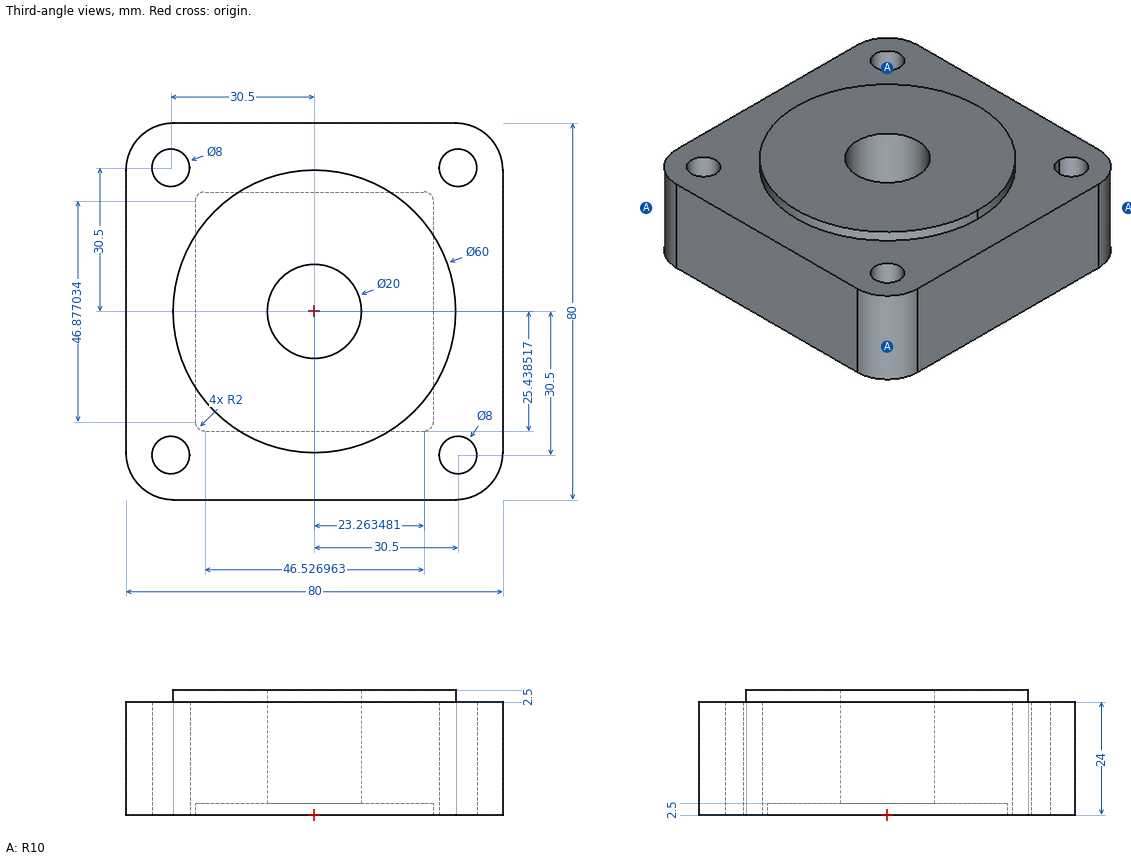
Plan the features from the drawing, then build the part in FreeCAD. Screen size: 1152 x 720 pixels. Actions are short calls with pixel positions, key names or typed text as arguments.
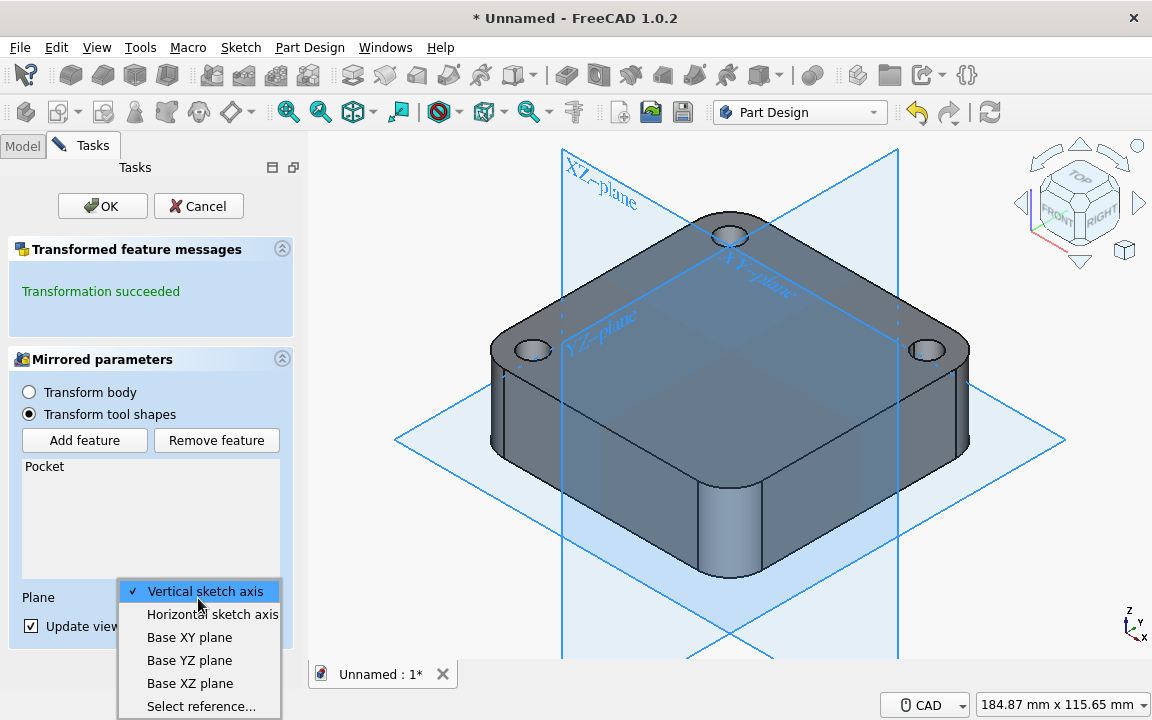
click(198, 660)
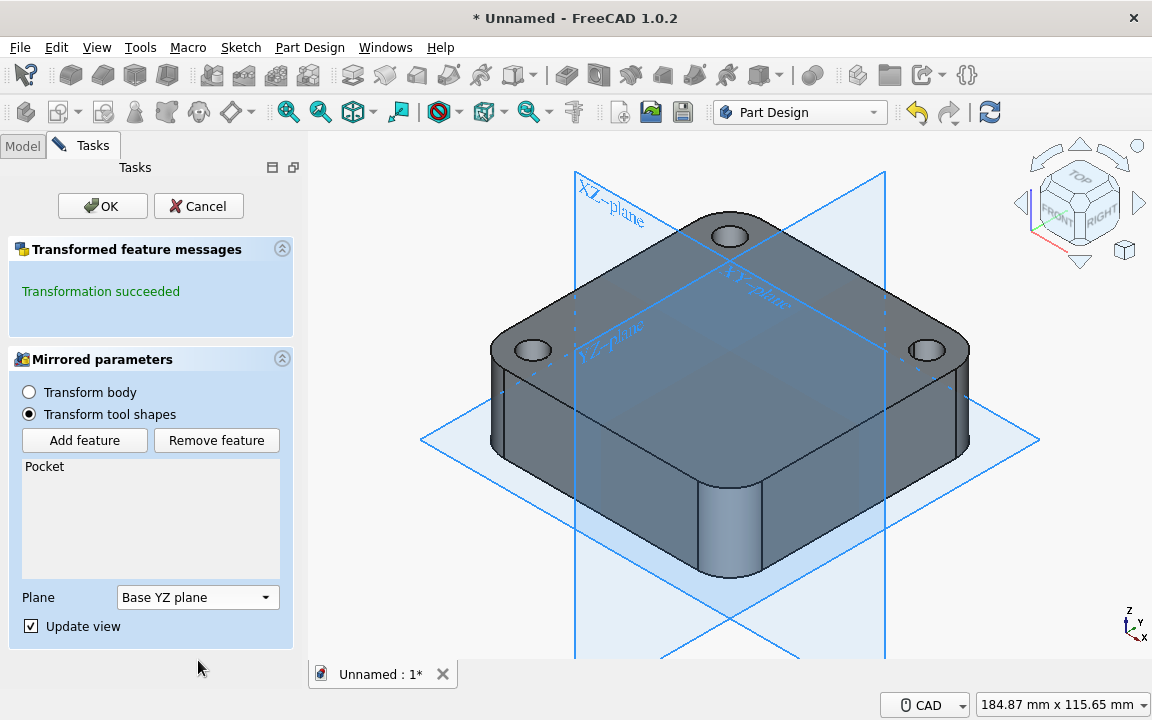
click(103, 206)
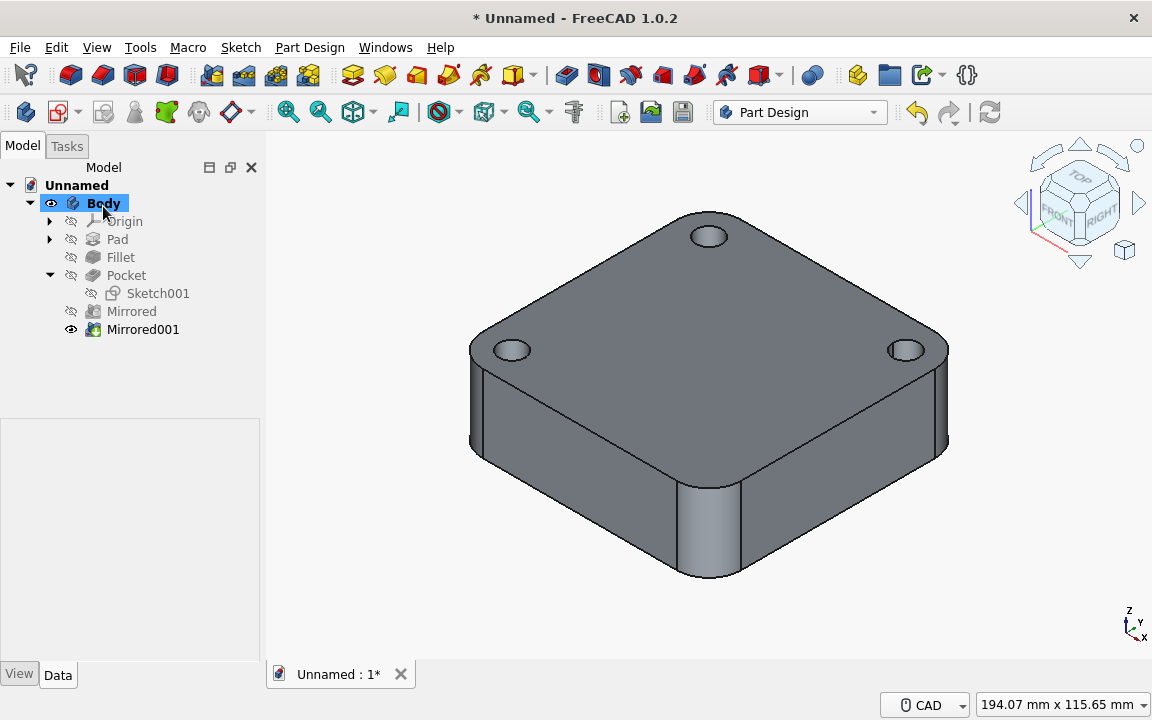
click(709, 349)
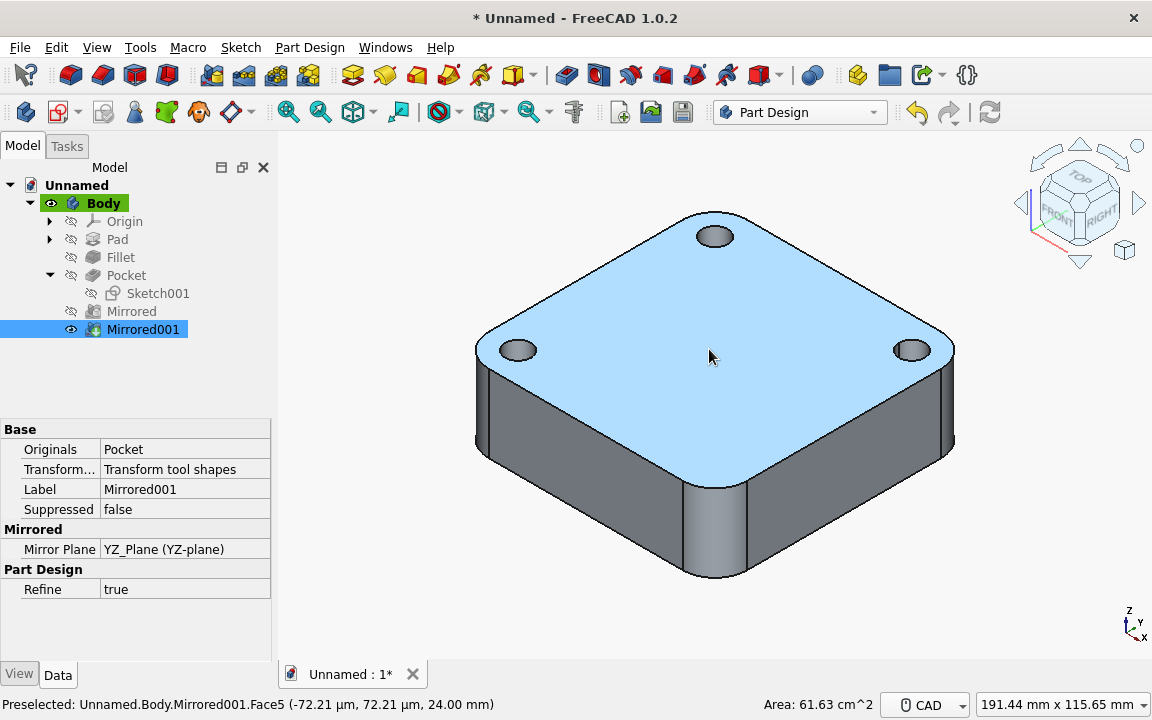
click(58, 112)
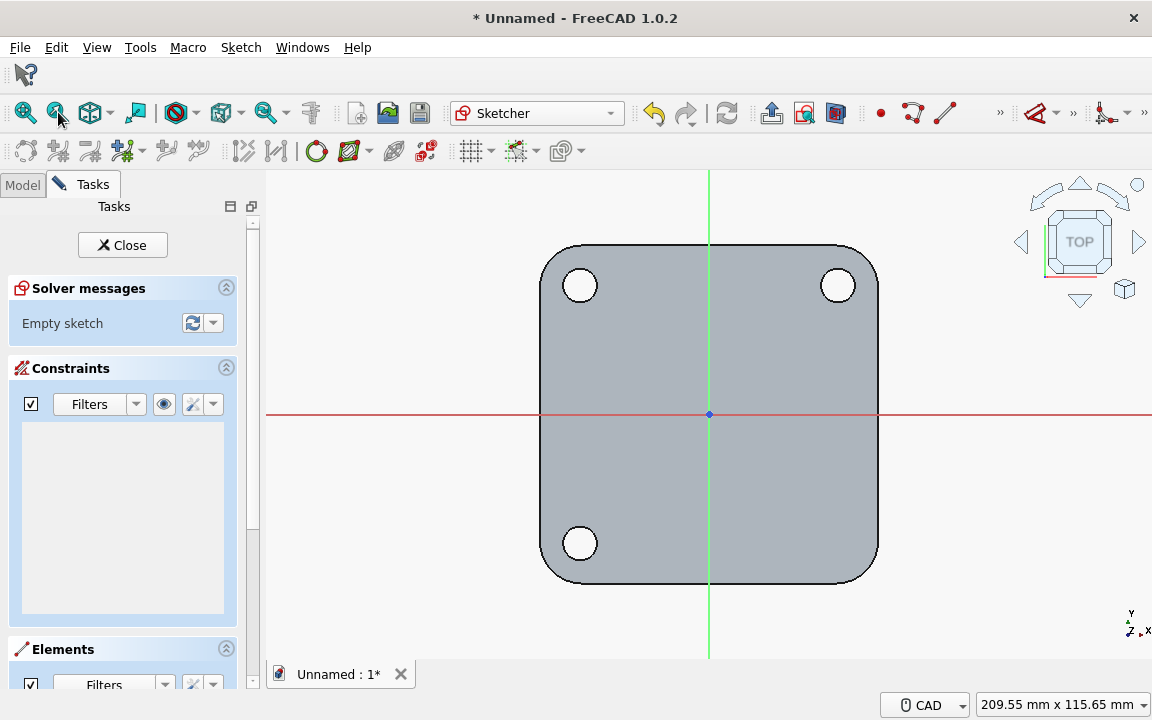
scroll(863, 560, up, 11)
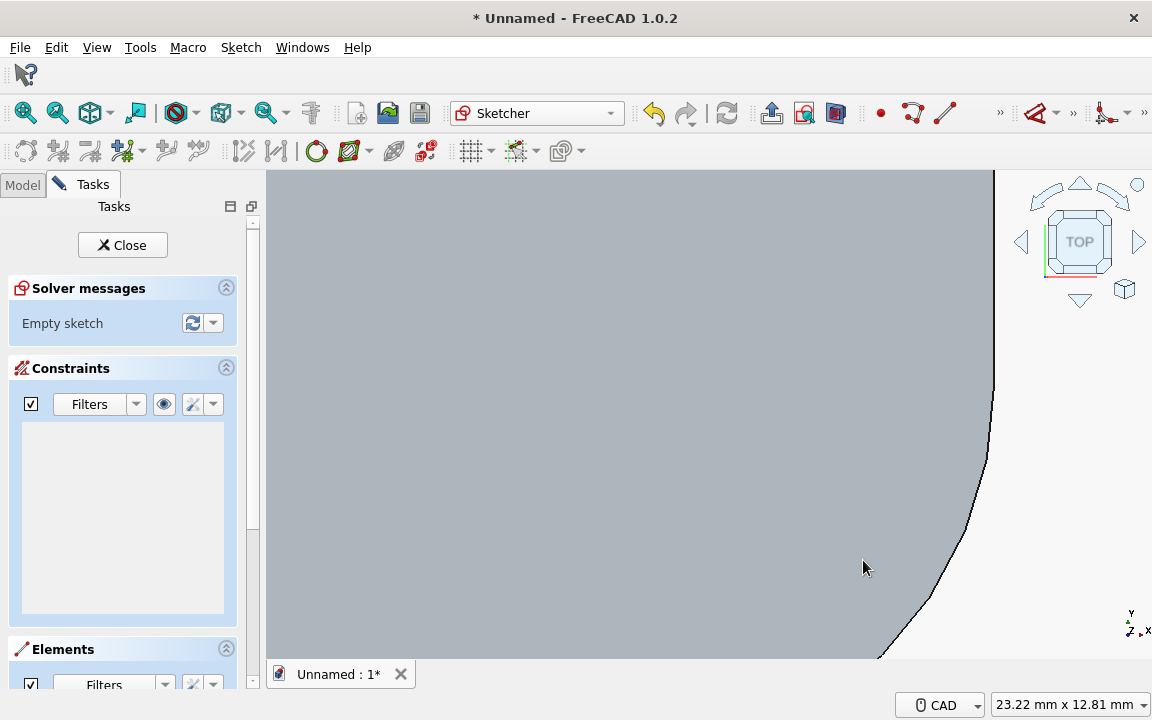
key(g)
key(c)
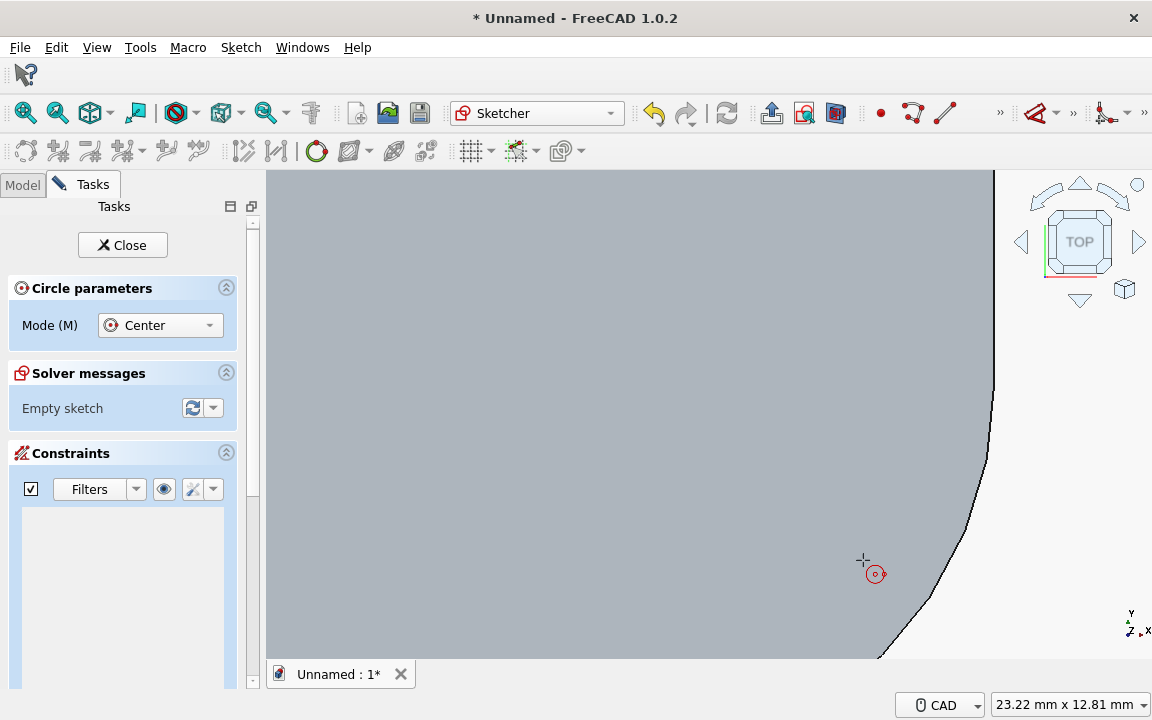
click(632, 404)
click(740, 296)
key(Escape)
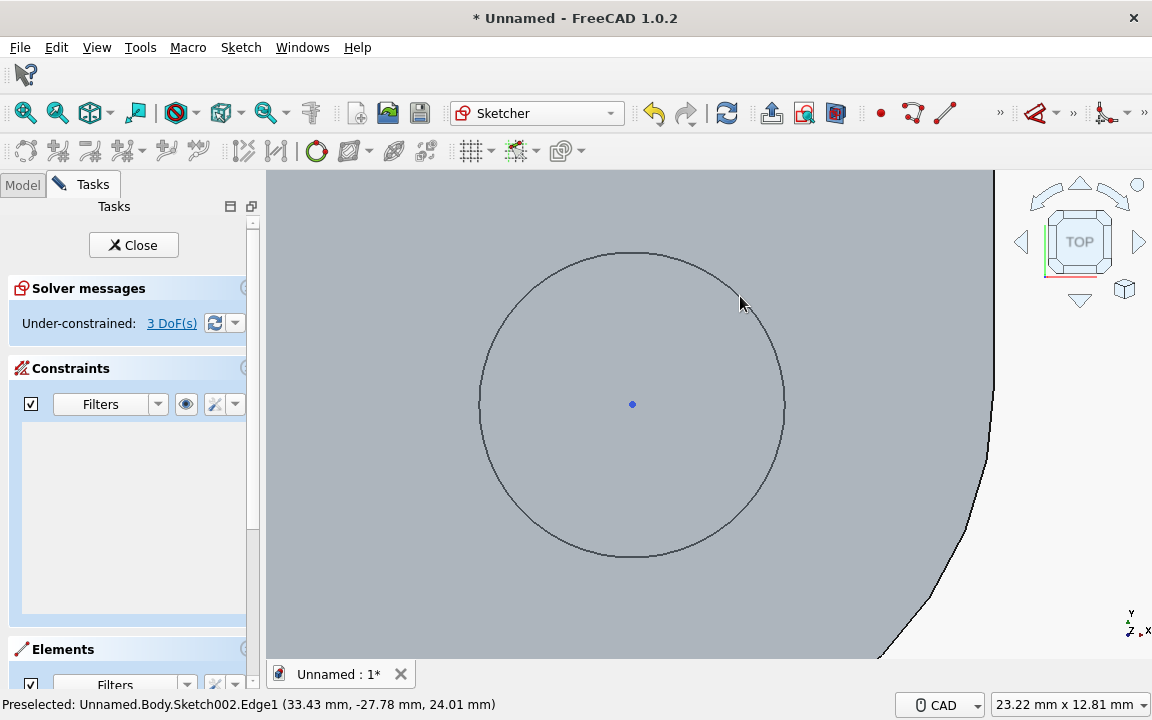
click(1036, 114)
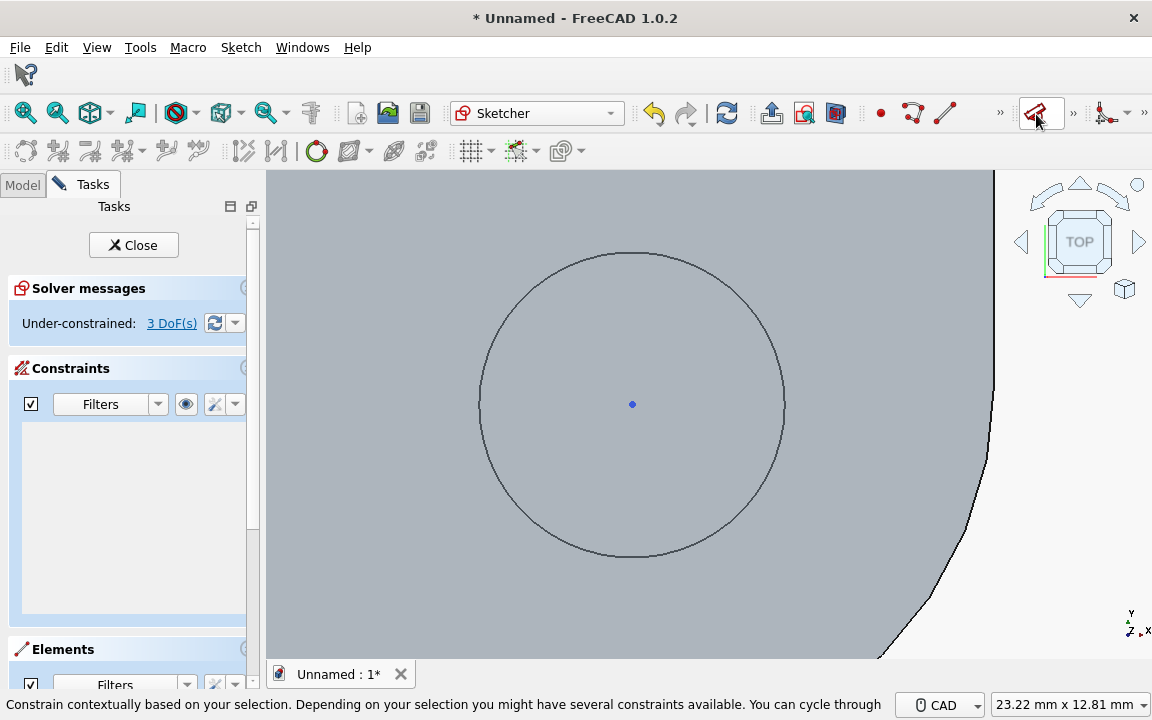
click(740, 297)
click(763, 274)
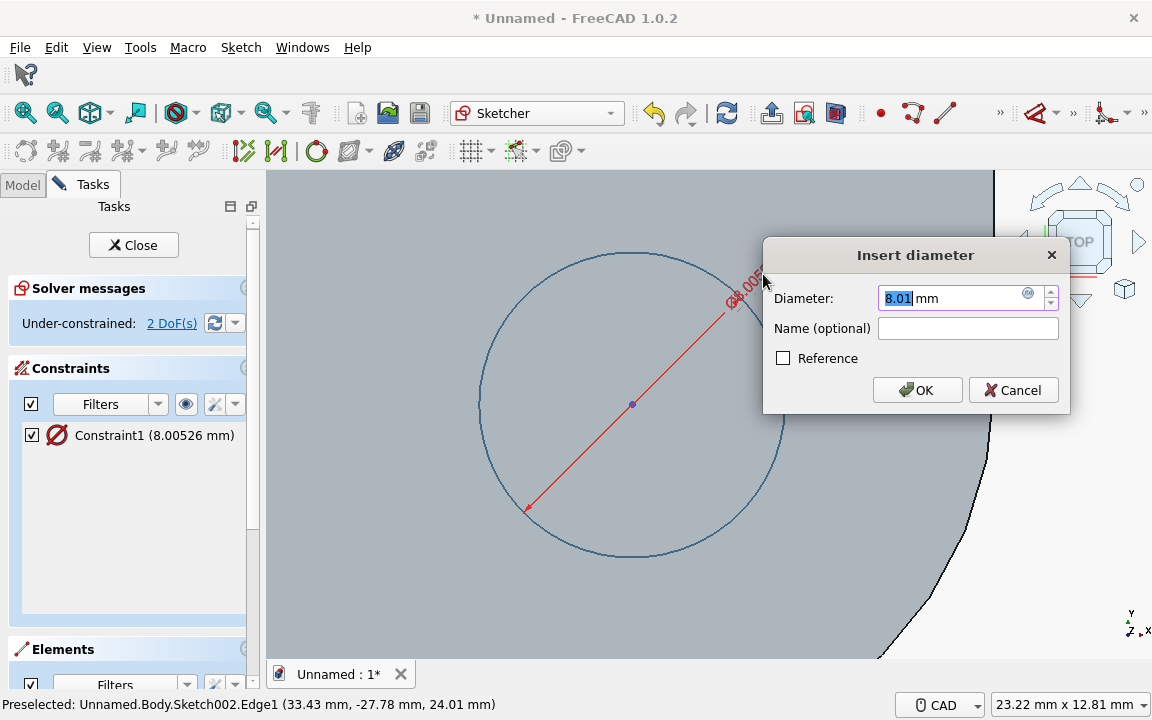
text(8)
key(Return)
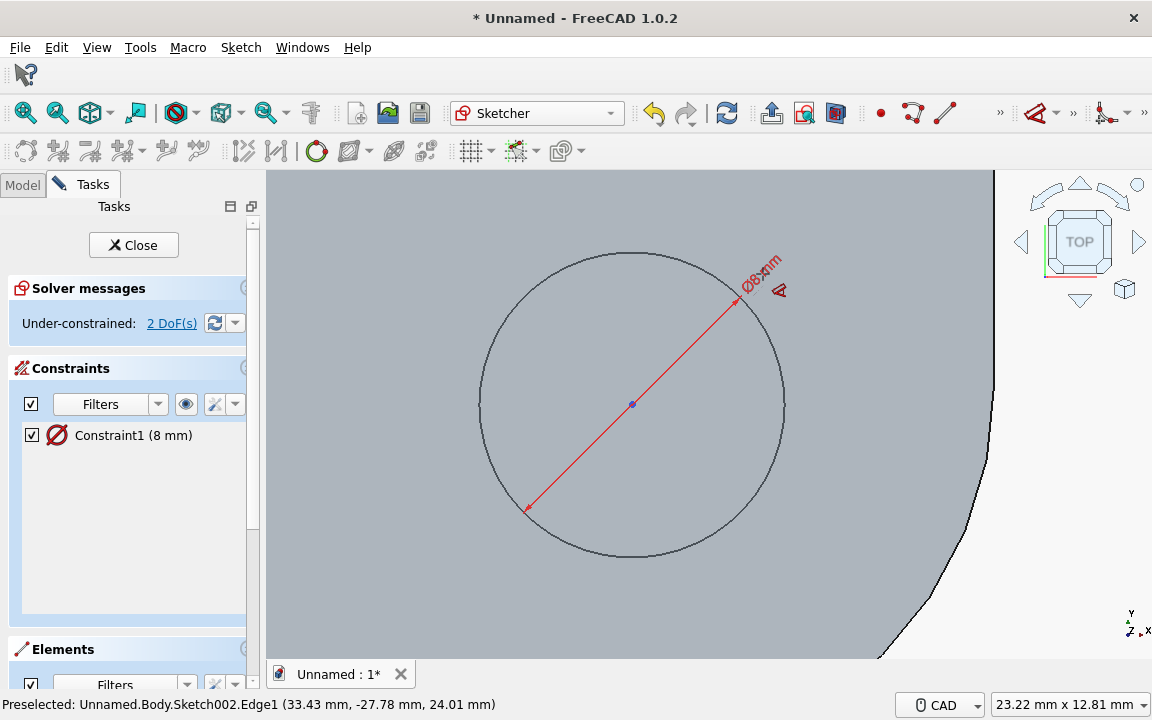
click(632, 405)
click(463, 439)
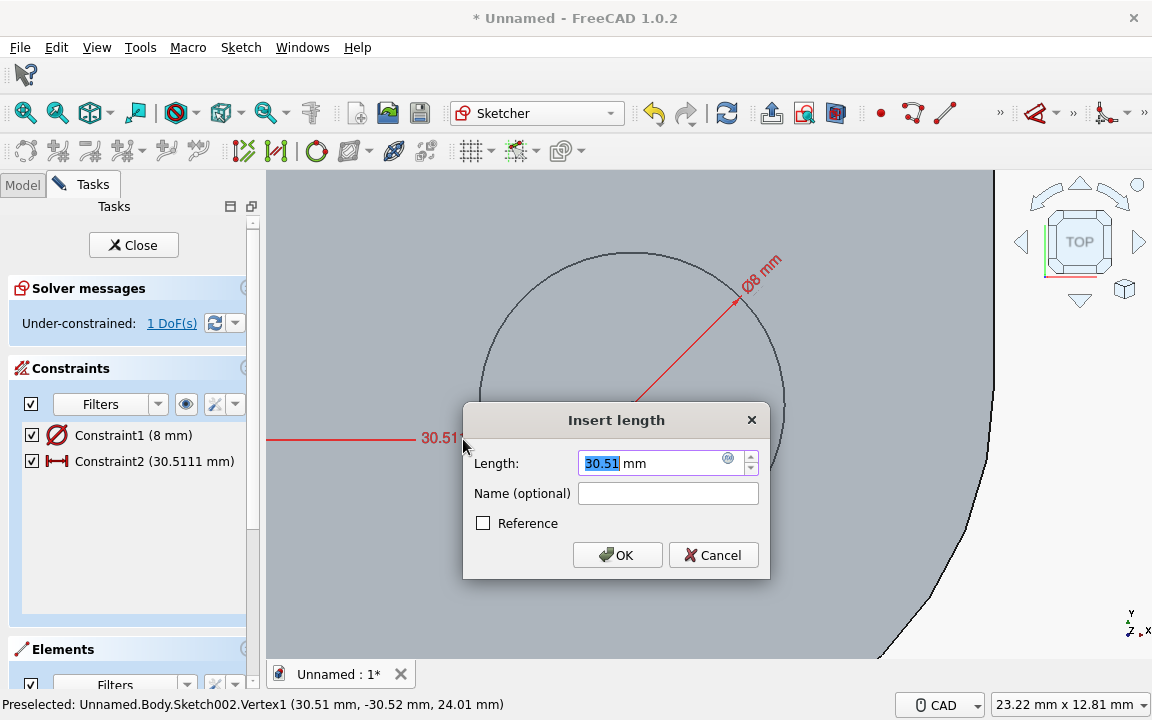
text(30.5)
key(Return)